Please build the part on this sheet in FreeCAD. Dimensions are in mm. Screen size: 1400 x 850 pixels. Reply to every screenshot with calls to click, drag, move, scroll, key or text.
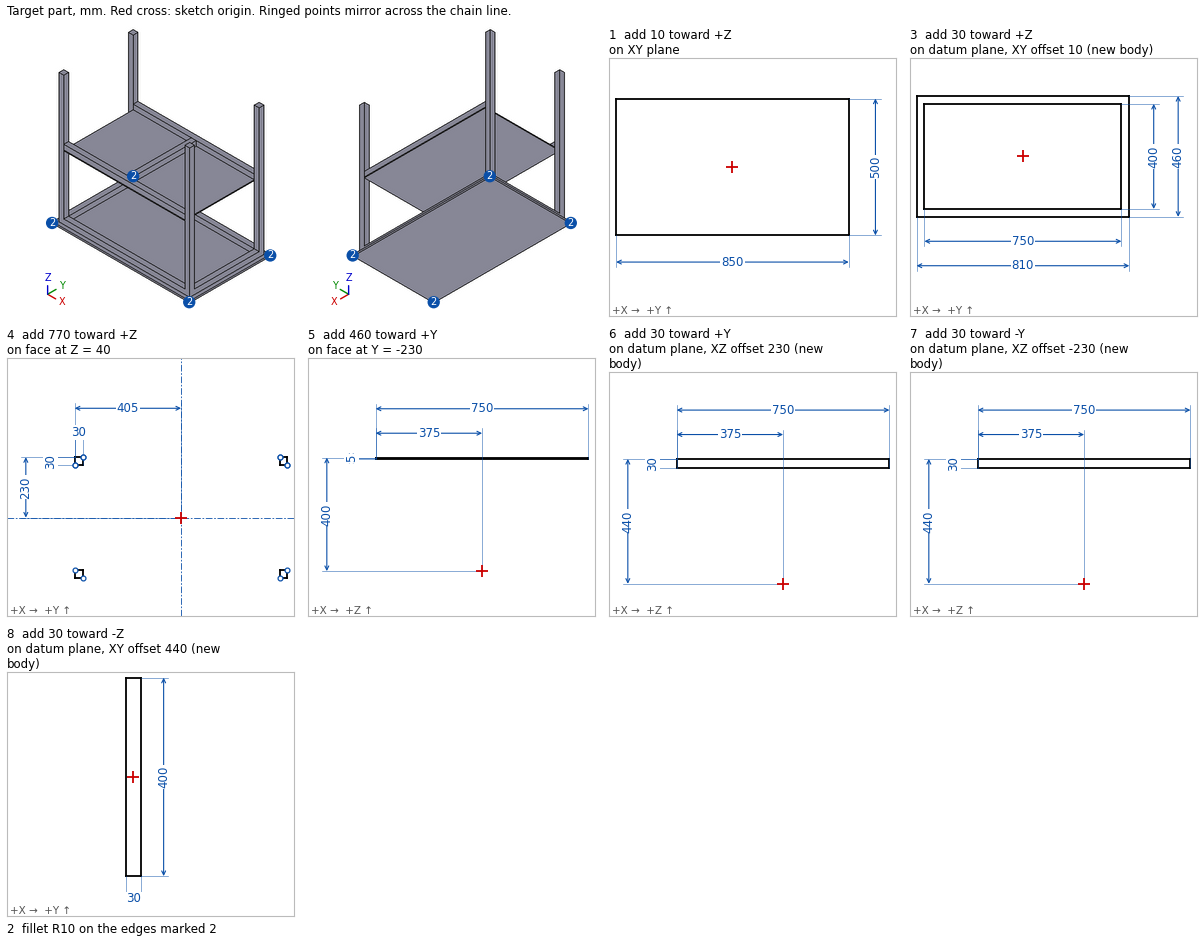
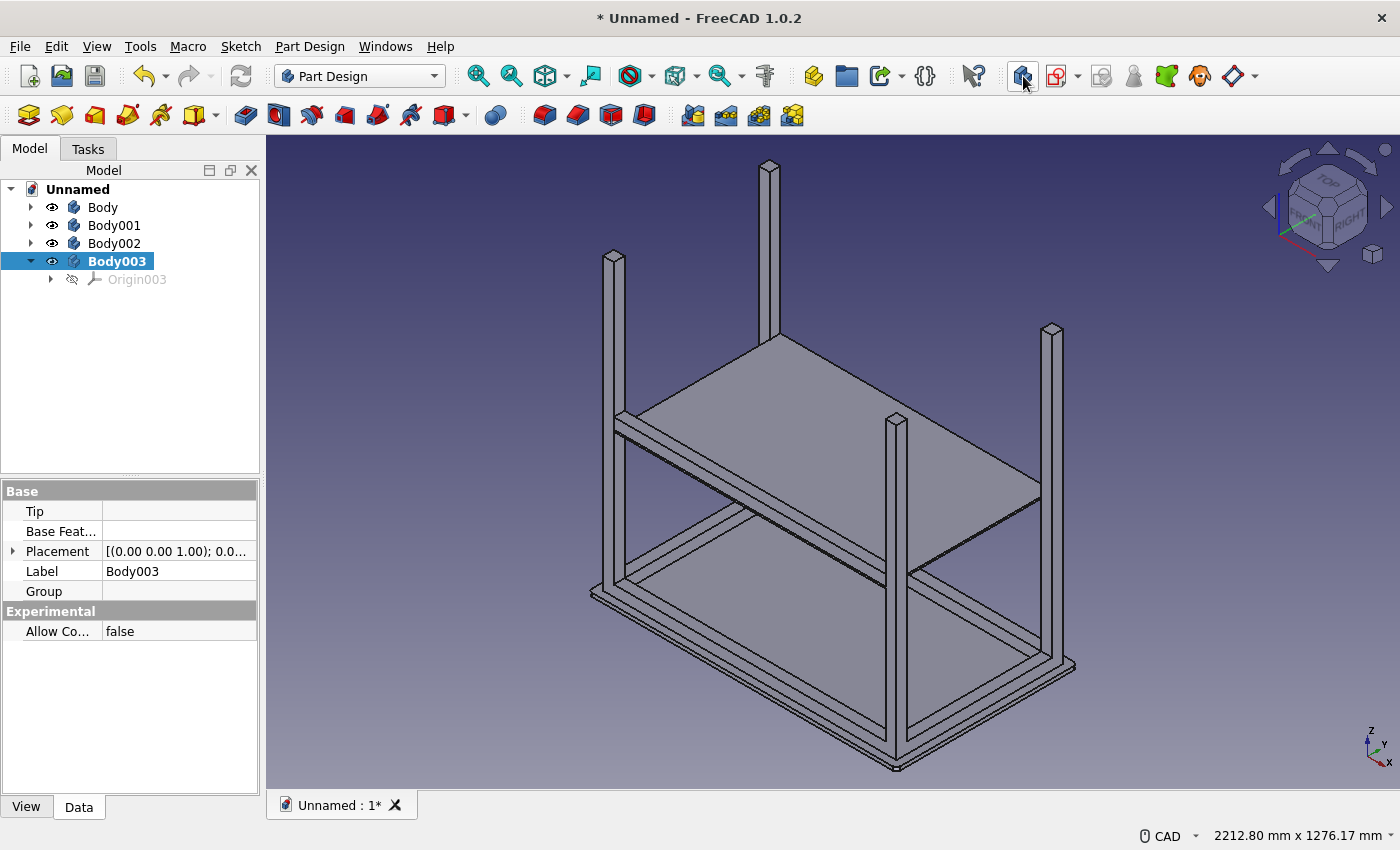
click(51, 279)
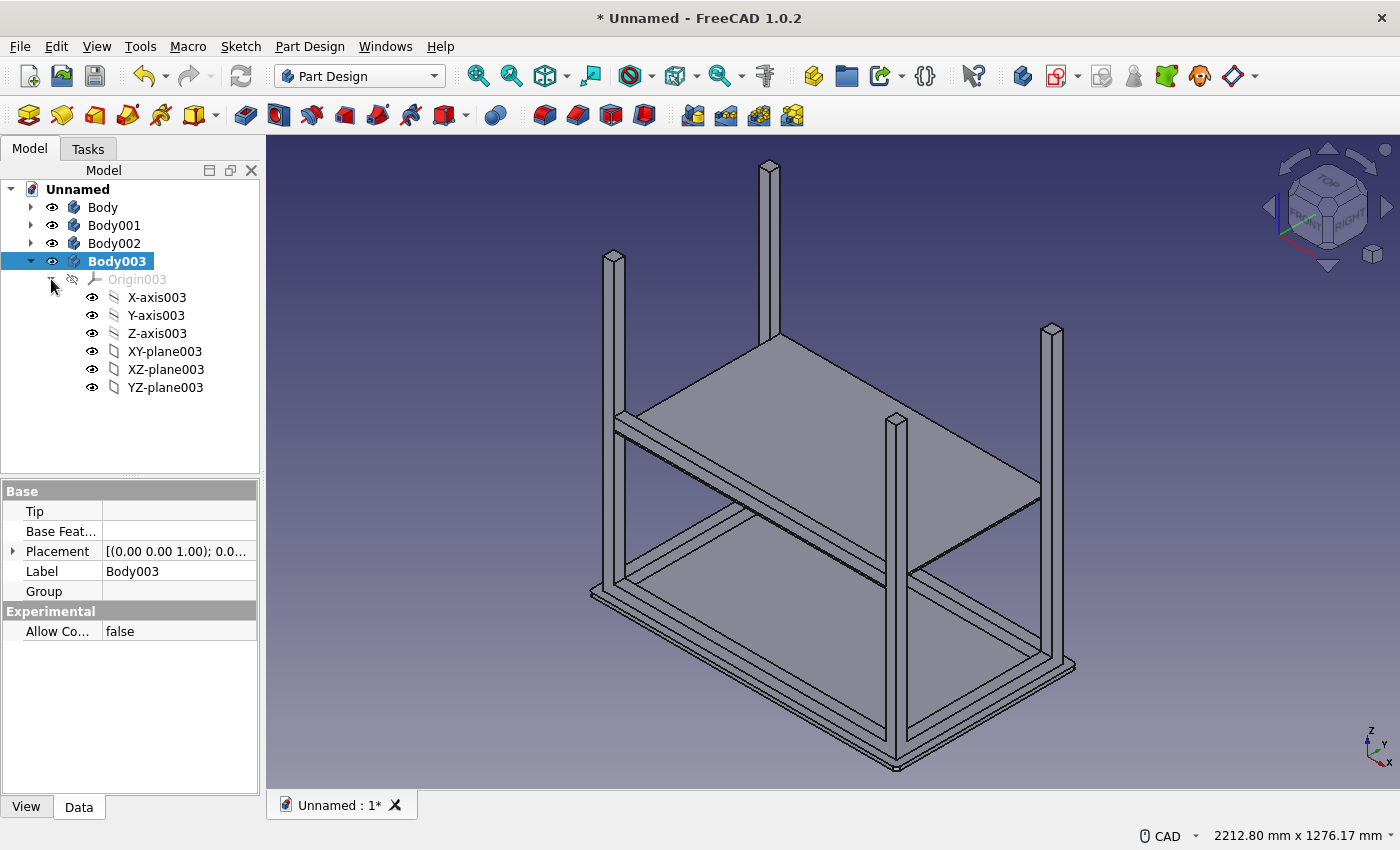
click(137, 369)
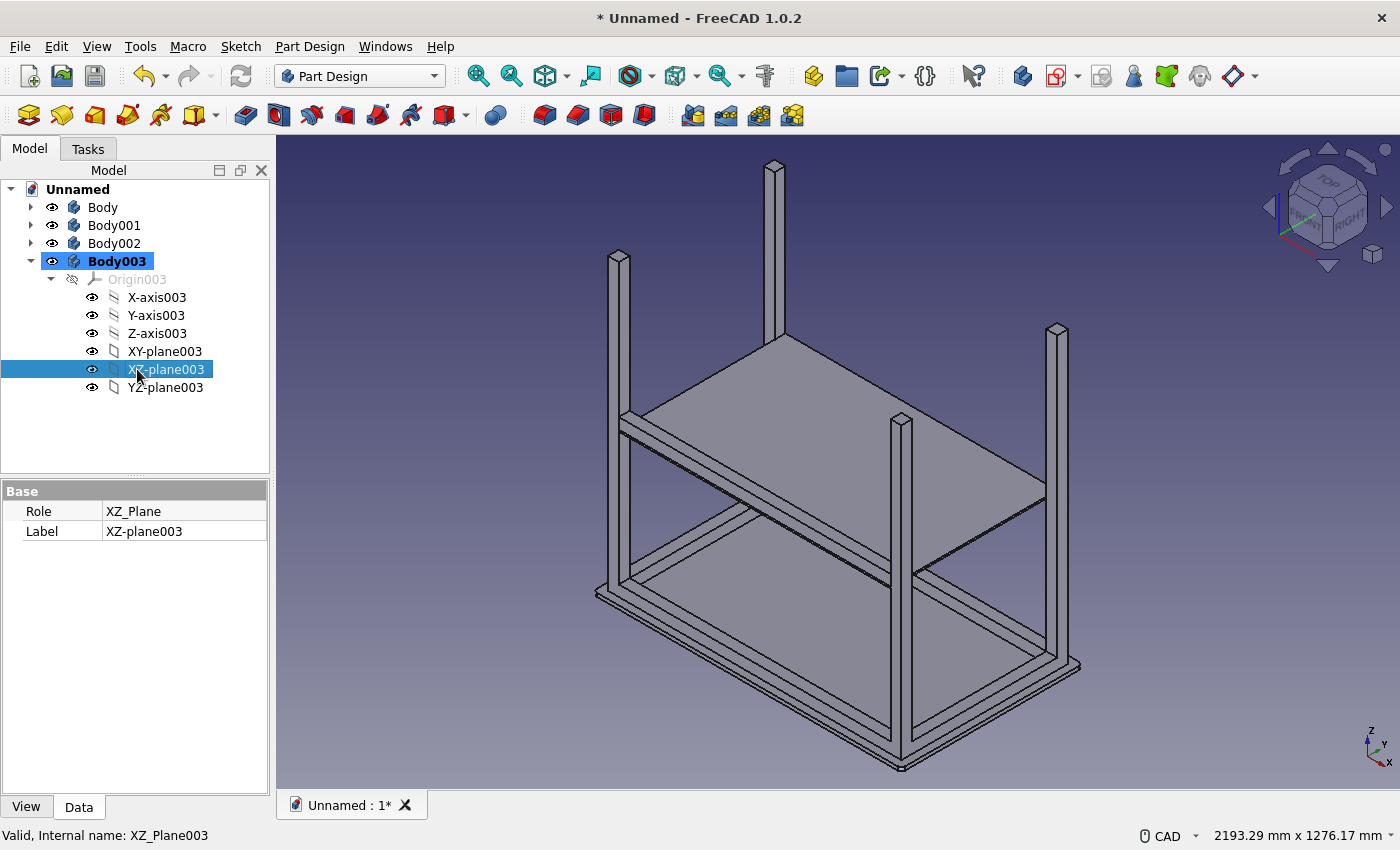
click(1232, 76)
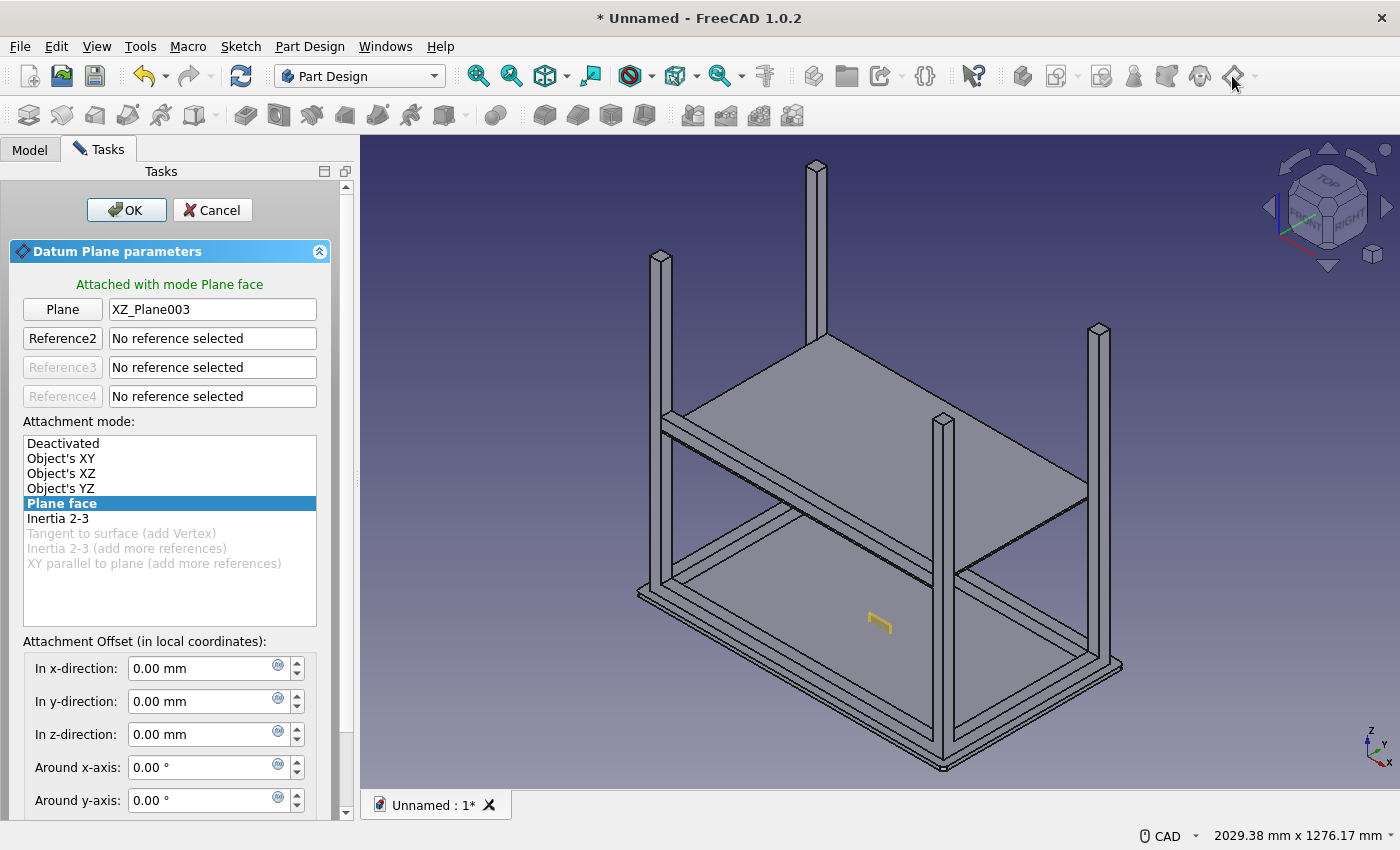
triple_click(210, 734)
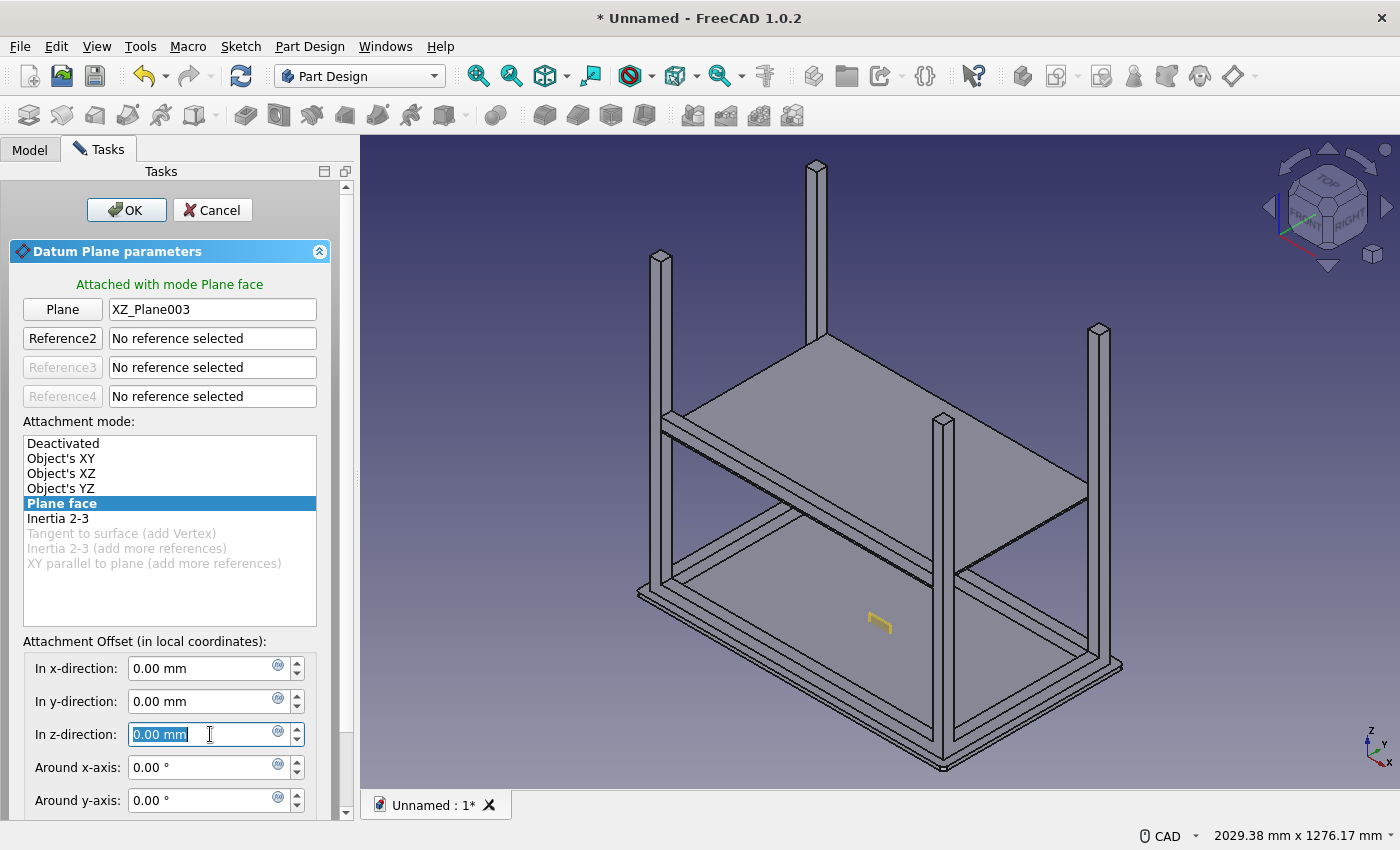
text(-230)
key(Tab)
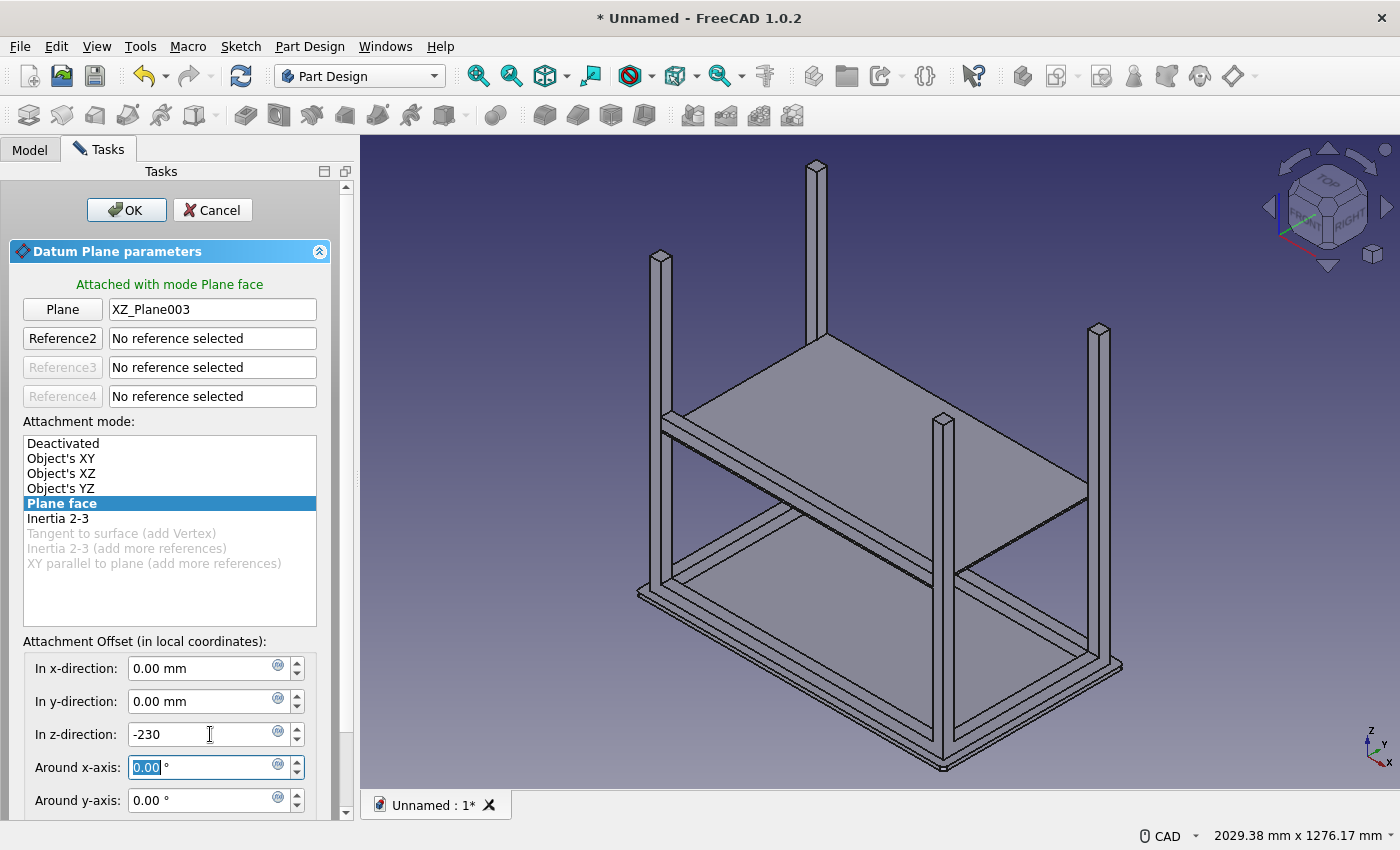
click(127, 210)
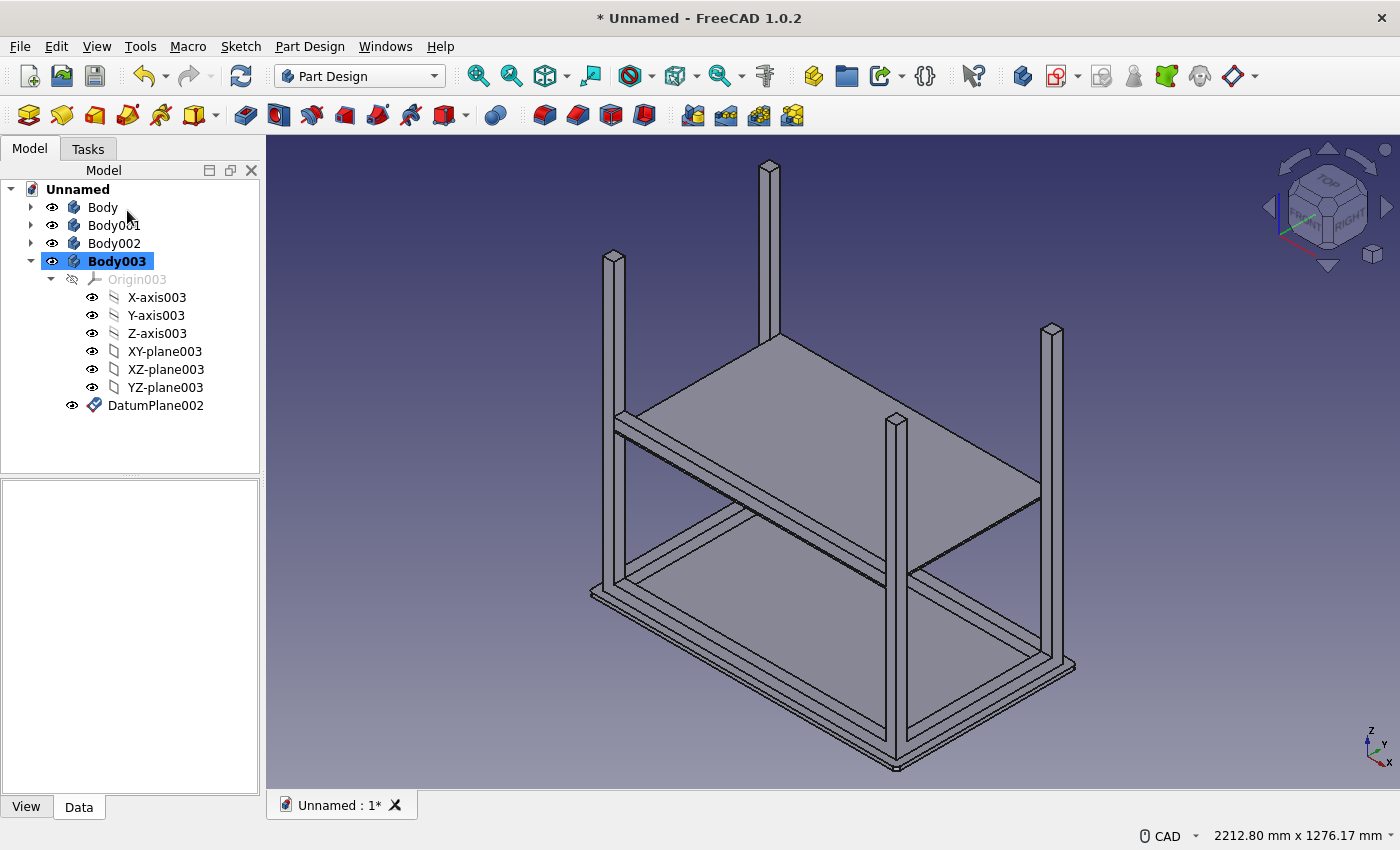
click(117, 405)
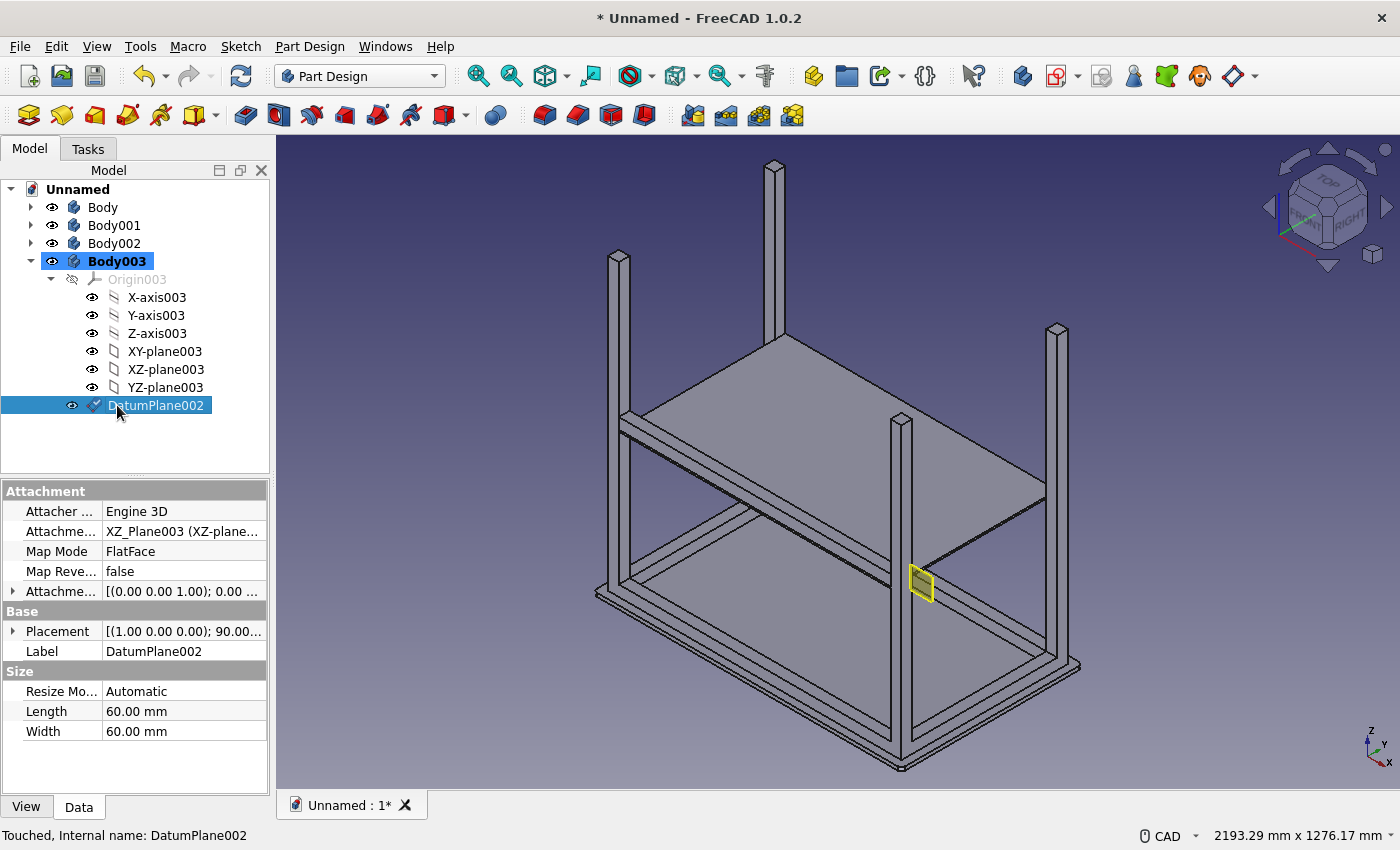
click(1056, 76)